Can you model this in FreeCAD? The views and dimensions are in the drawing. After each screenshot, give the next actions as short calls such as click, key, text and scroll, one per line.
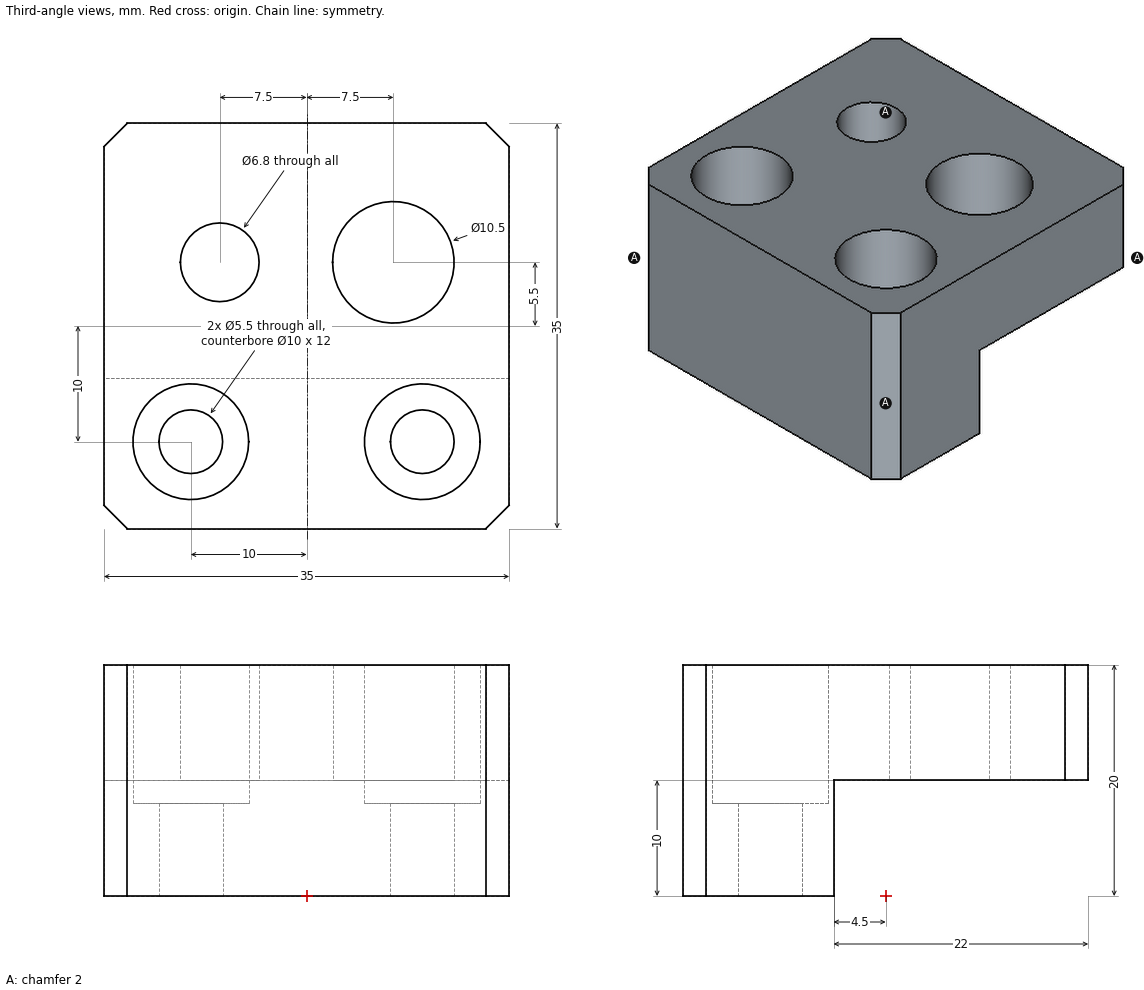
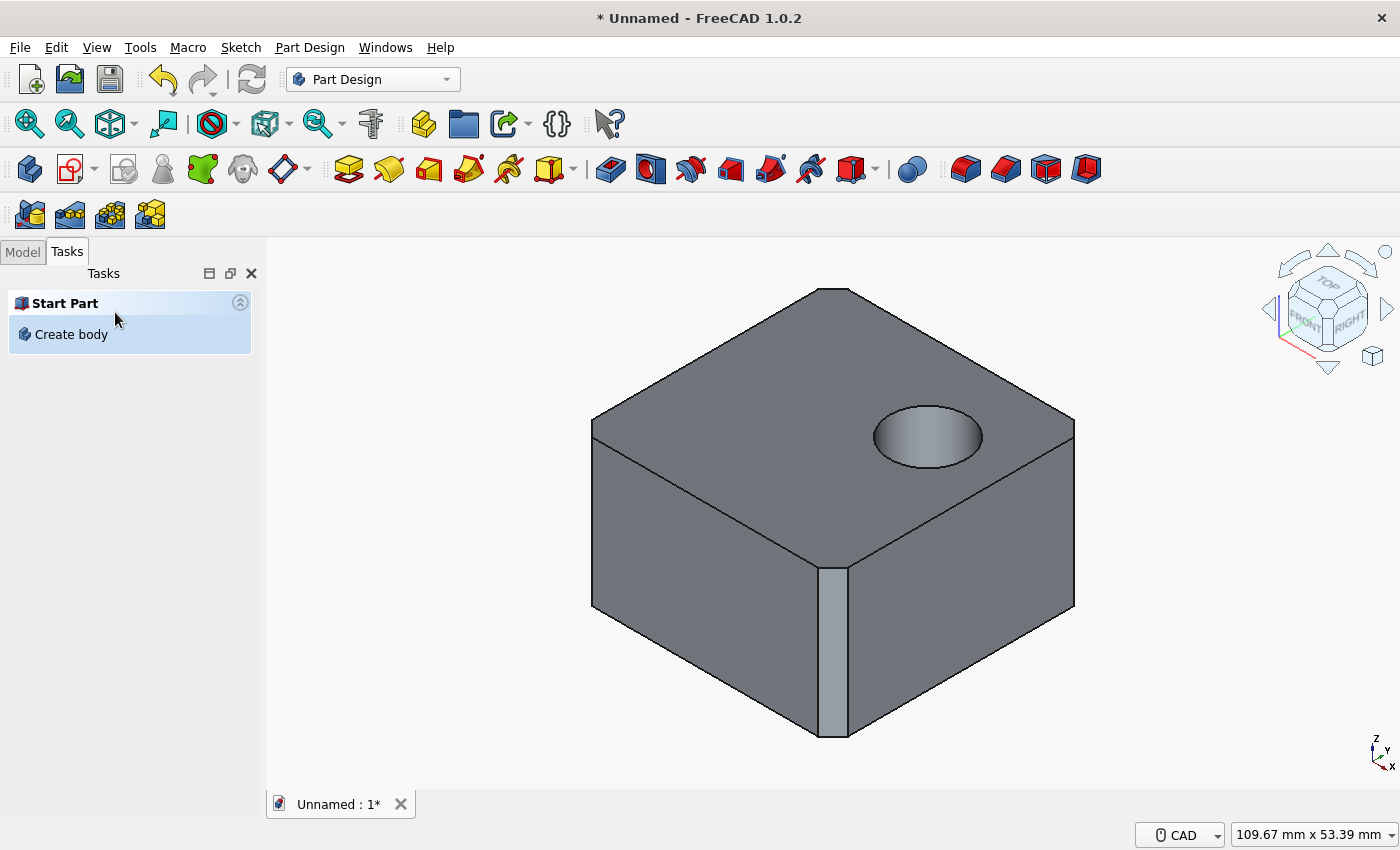
click(760, 428)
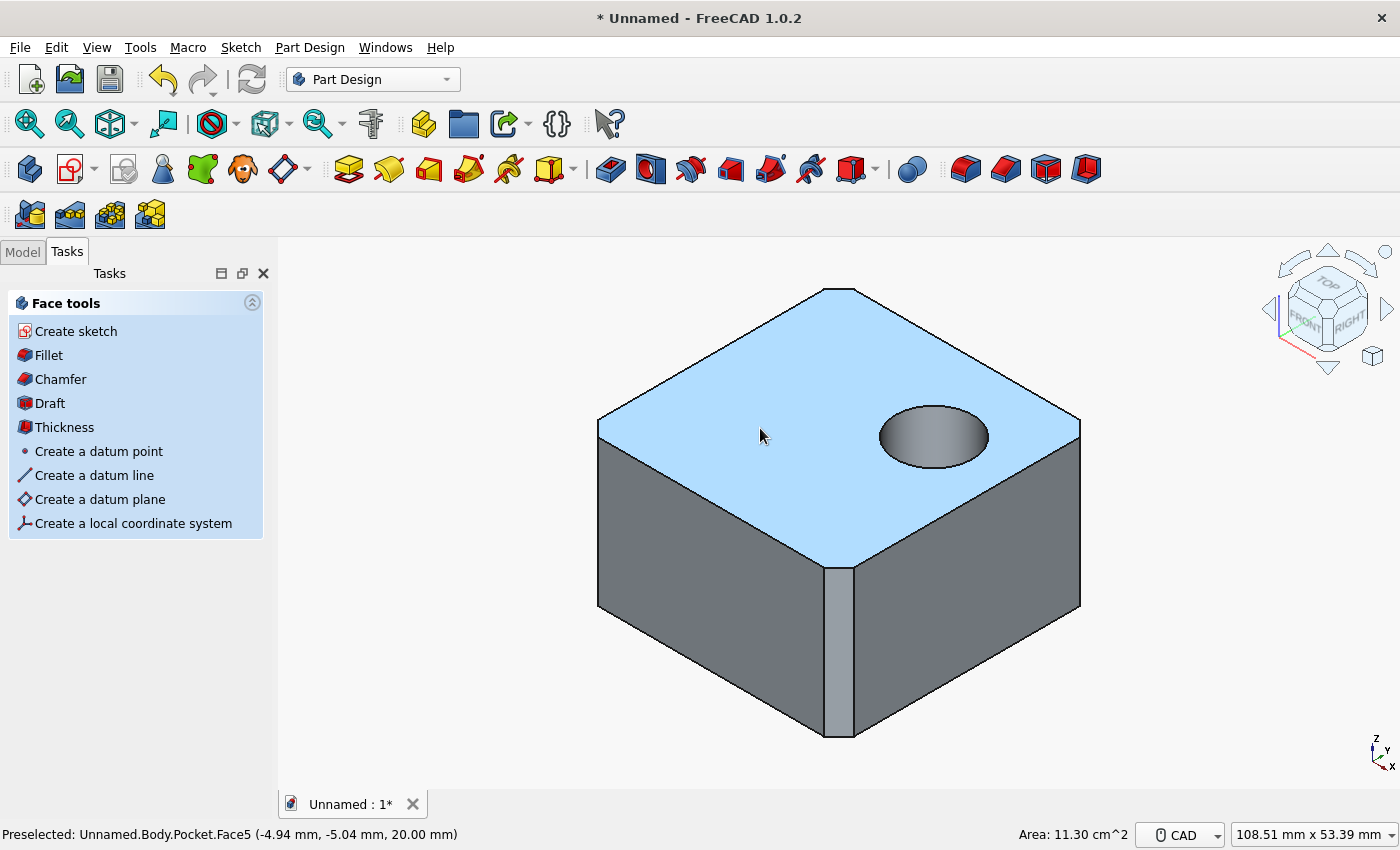
click(70, 170)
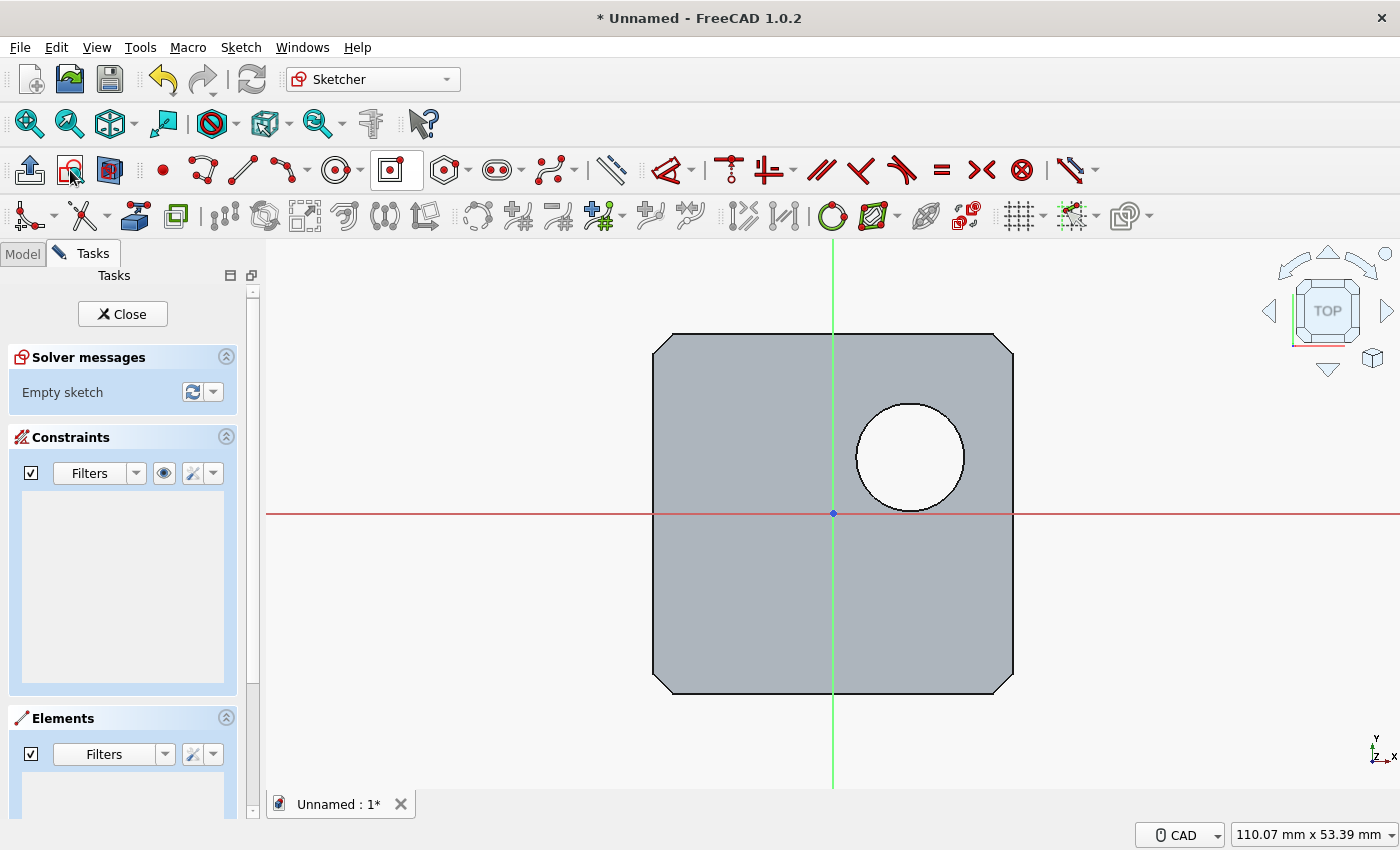
scroll(781, 453, up, 7)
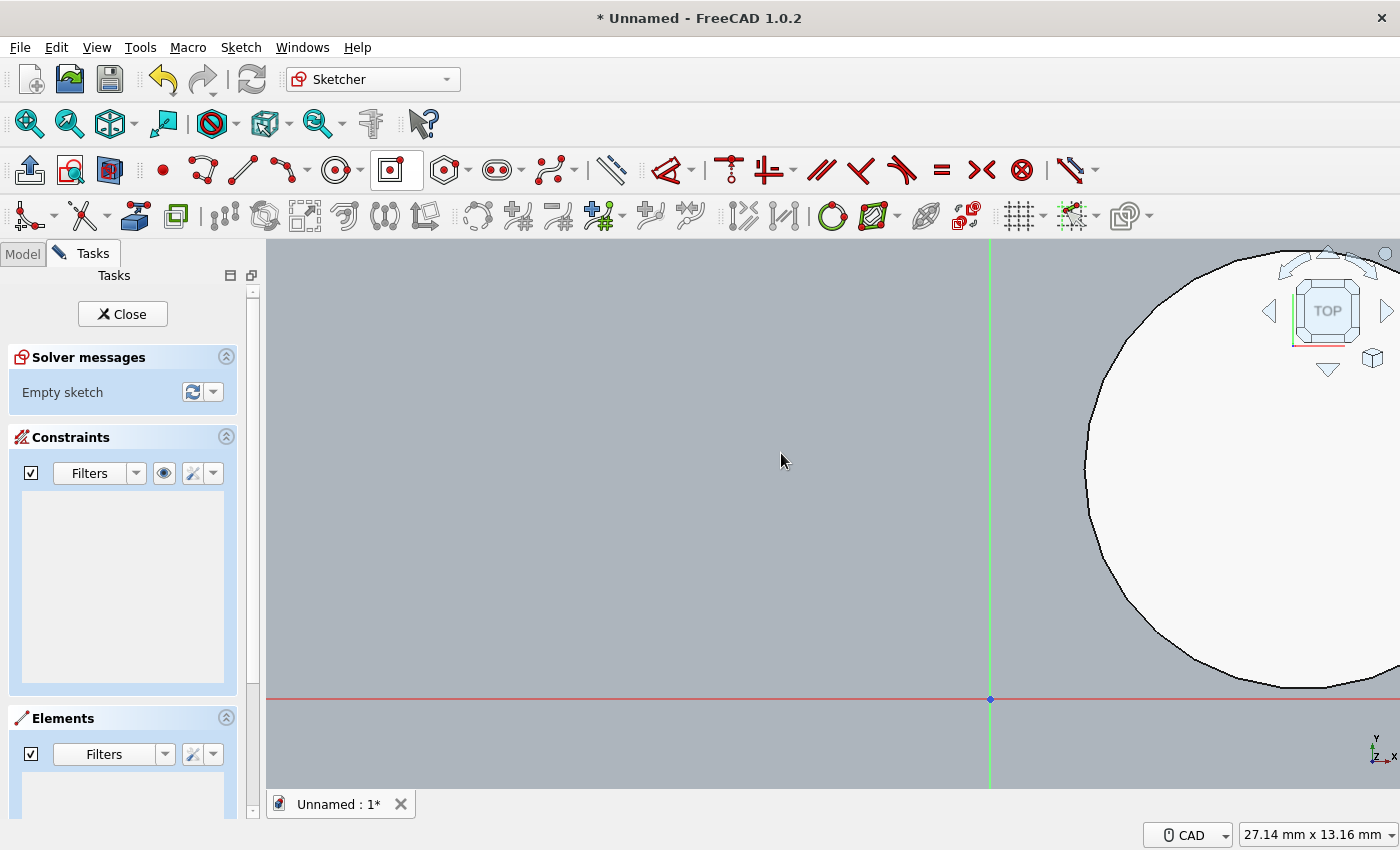
key(g)
key(c)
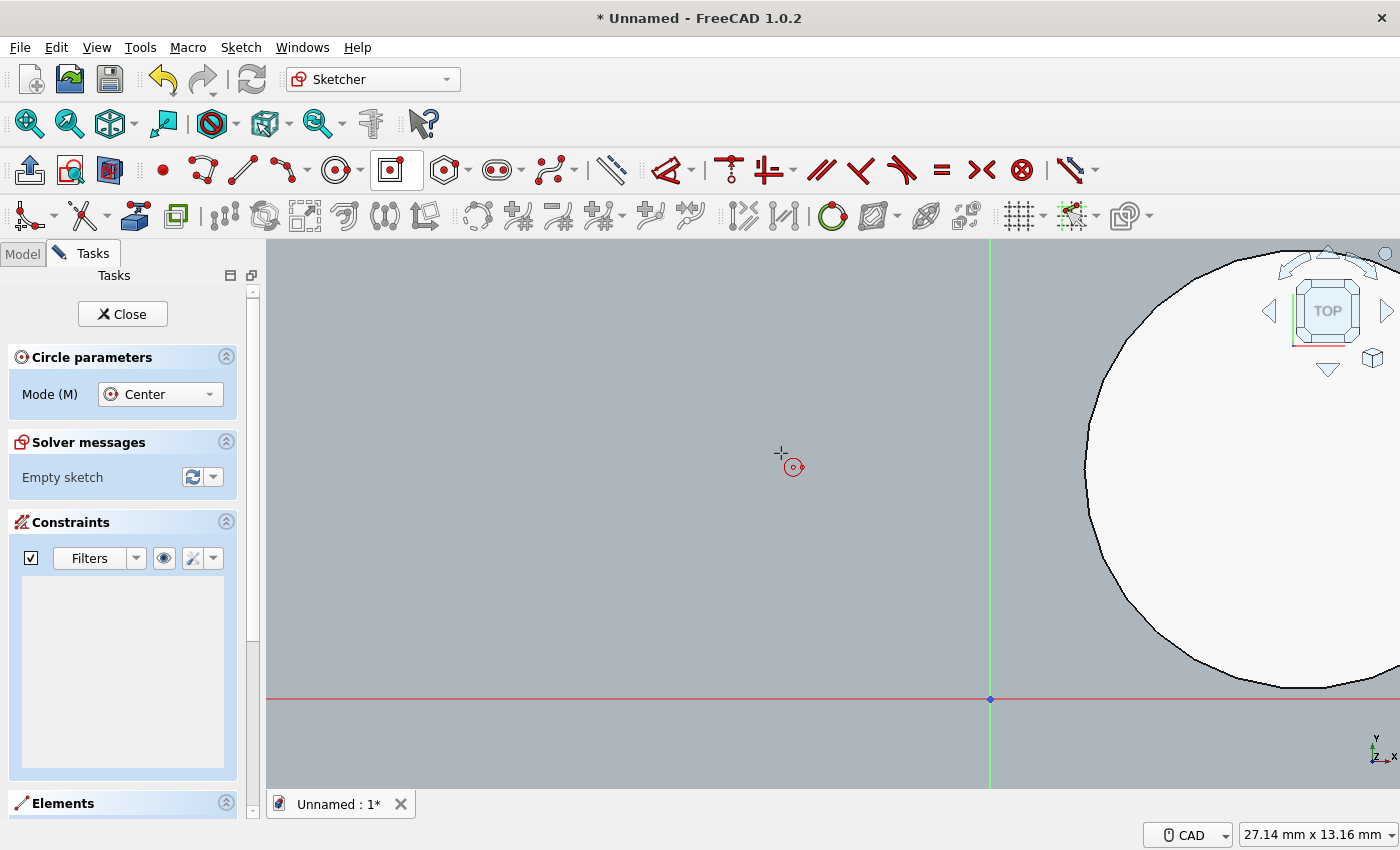
click(677, 469)
move(778, 369)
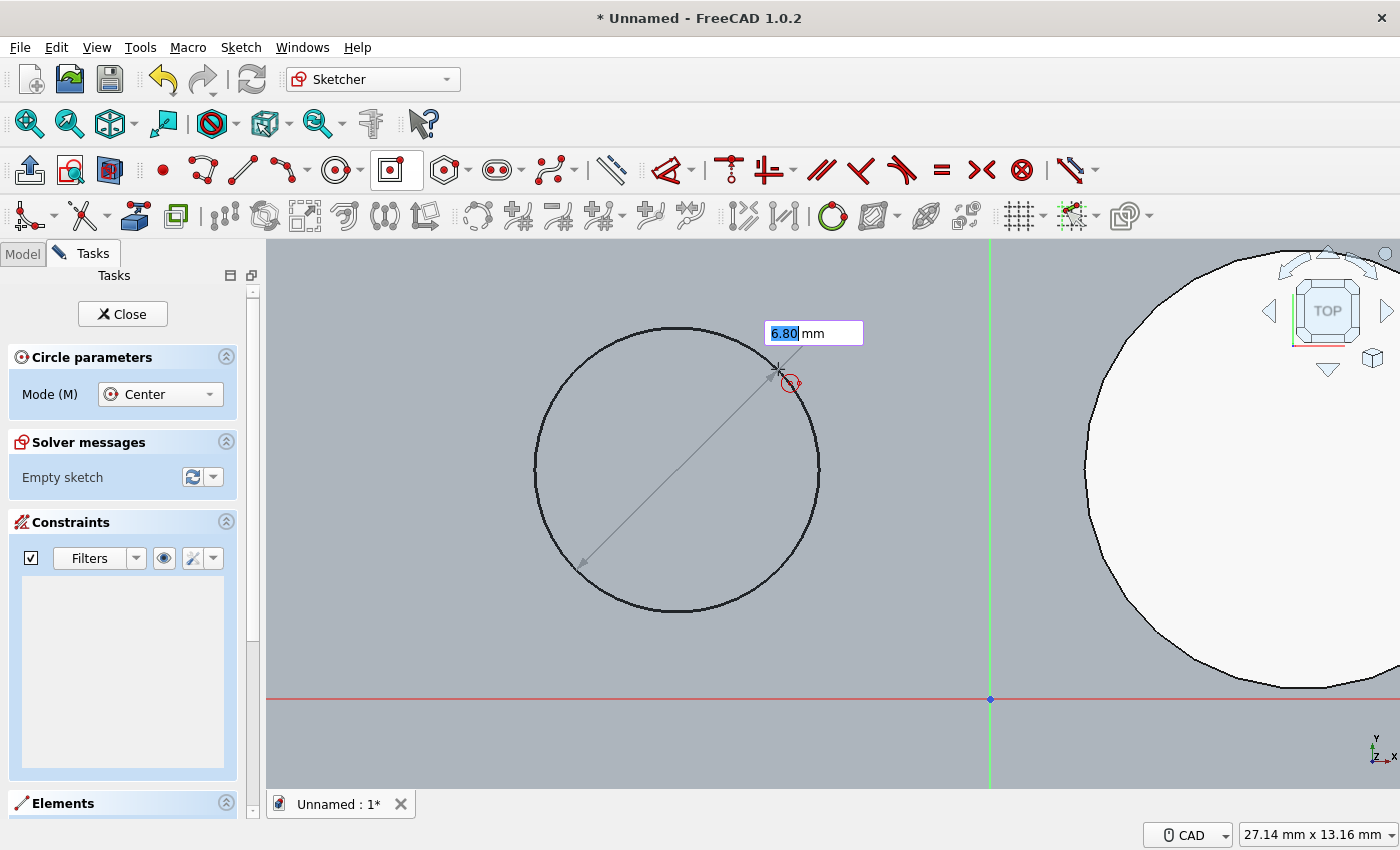
text(6.8)
key(Return)
key(Escape)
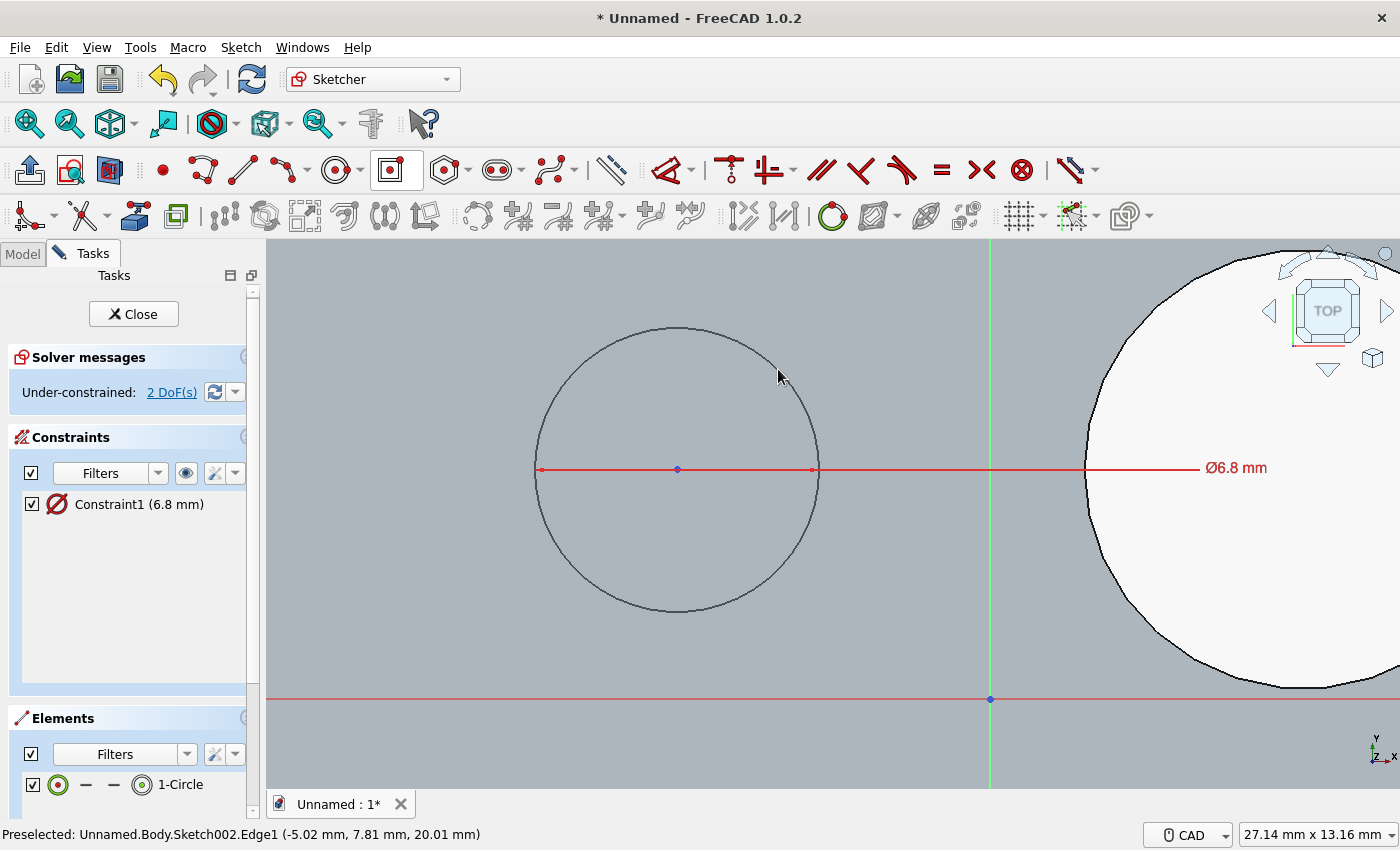
click(666, 170)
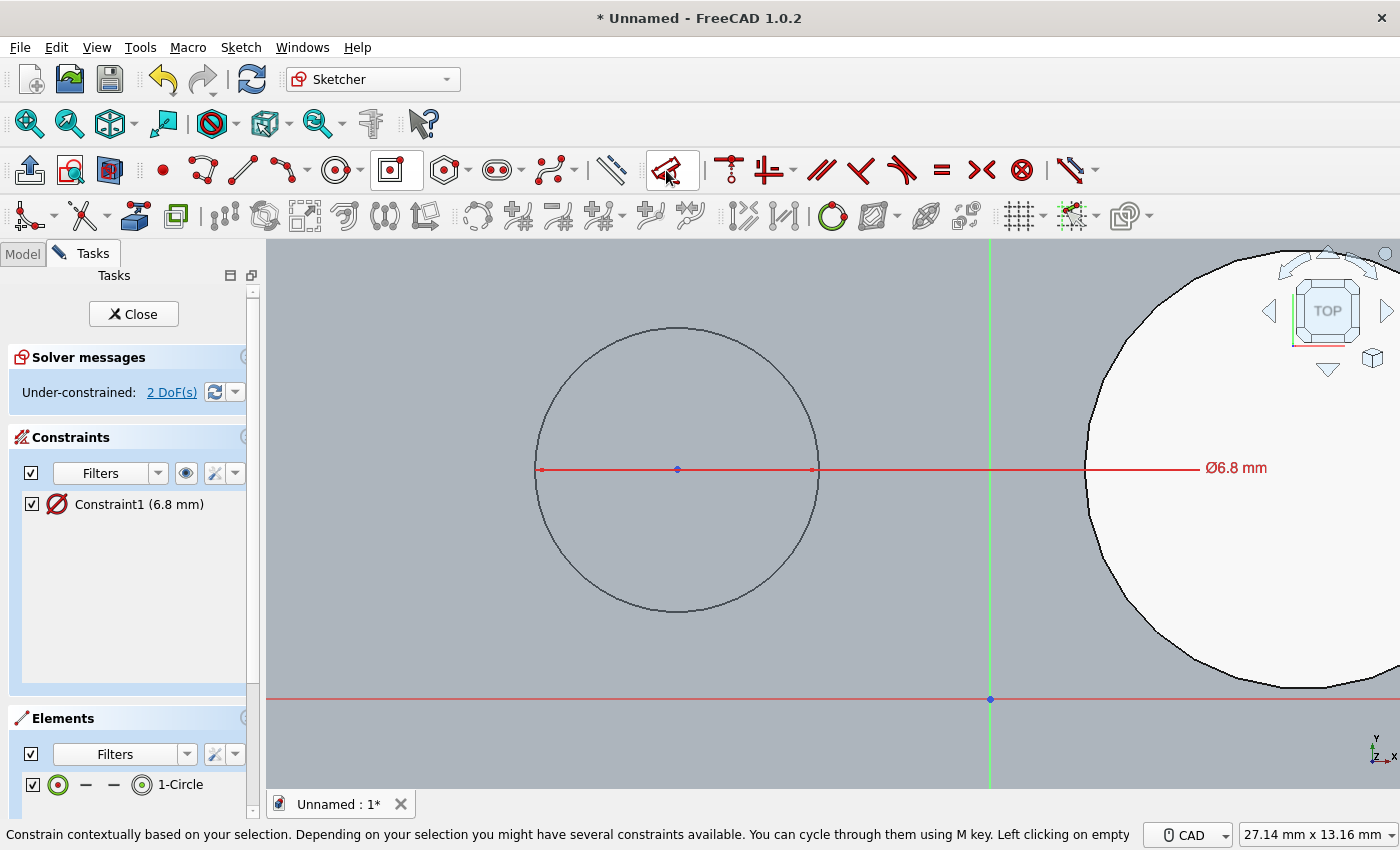
click(677, 470)
click(834, 733)